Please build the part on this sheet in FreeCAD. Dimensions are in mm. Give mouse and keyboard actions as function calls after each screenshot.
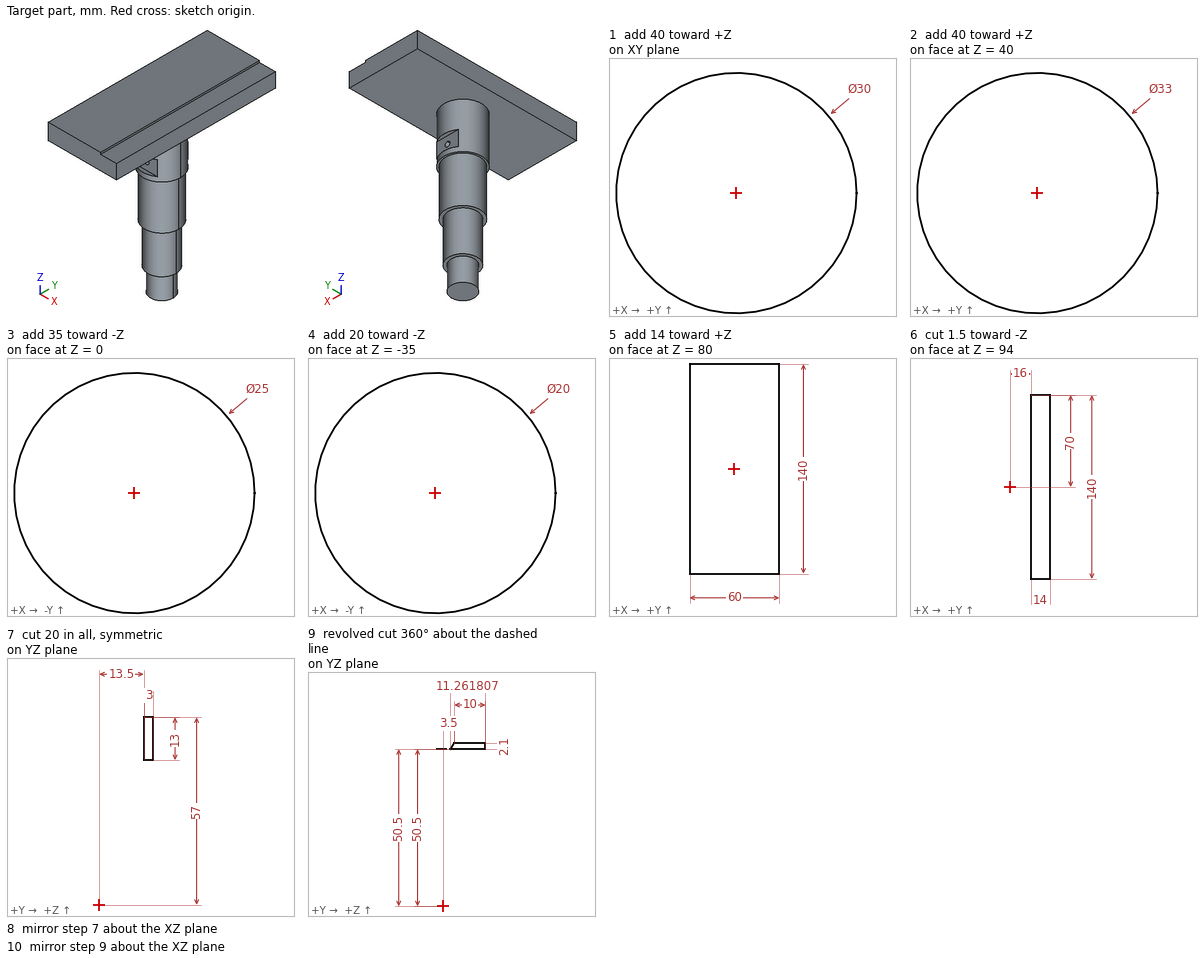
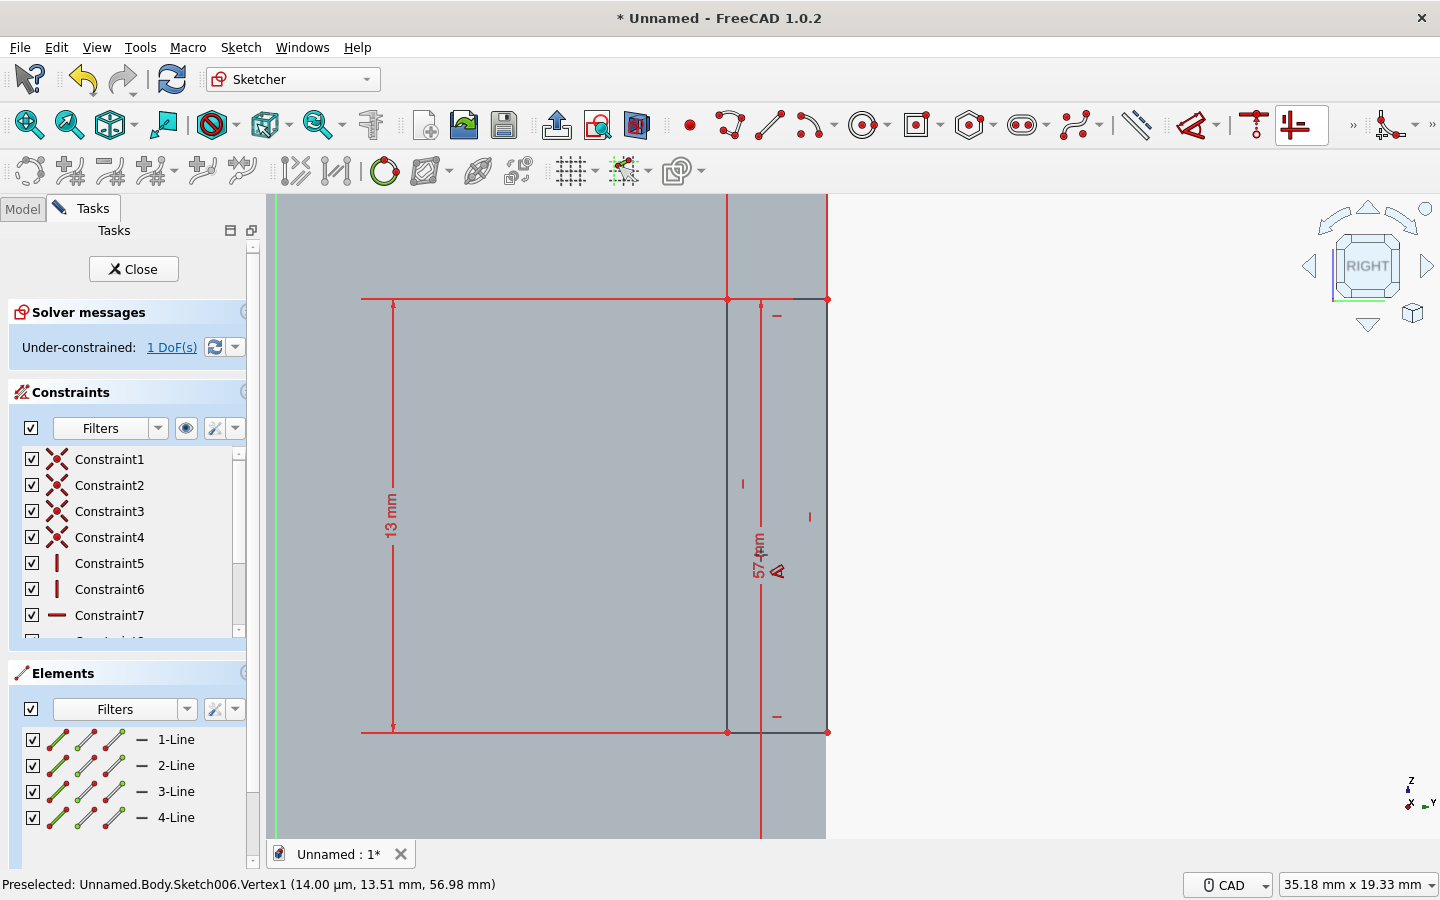
click(727, 299)
click(511, 265)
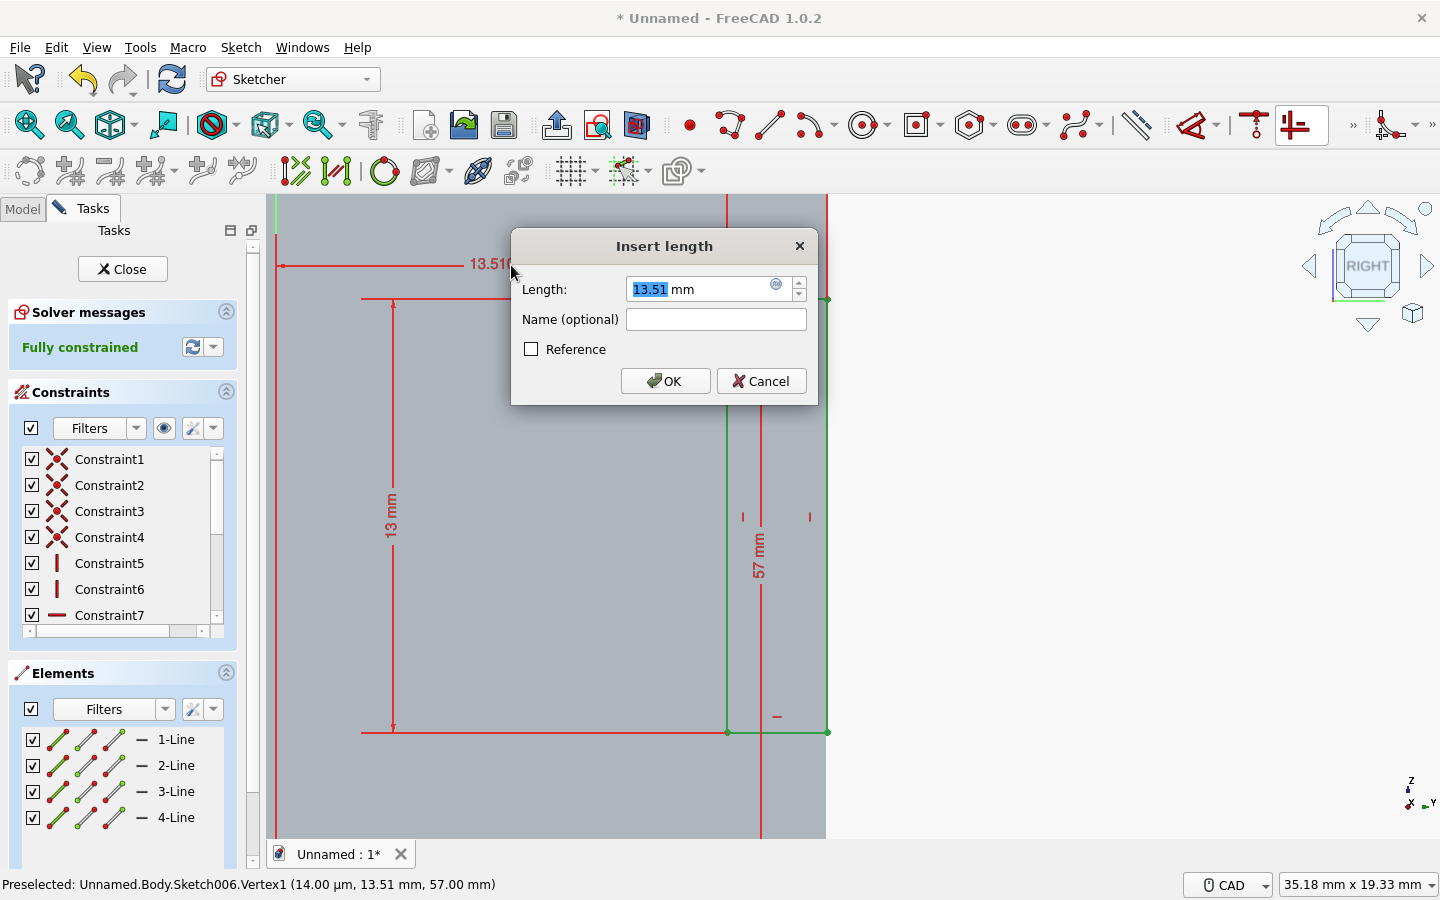
text(13.5)
key(Return)
key(Escape)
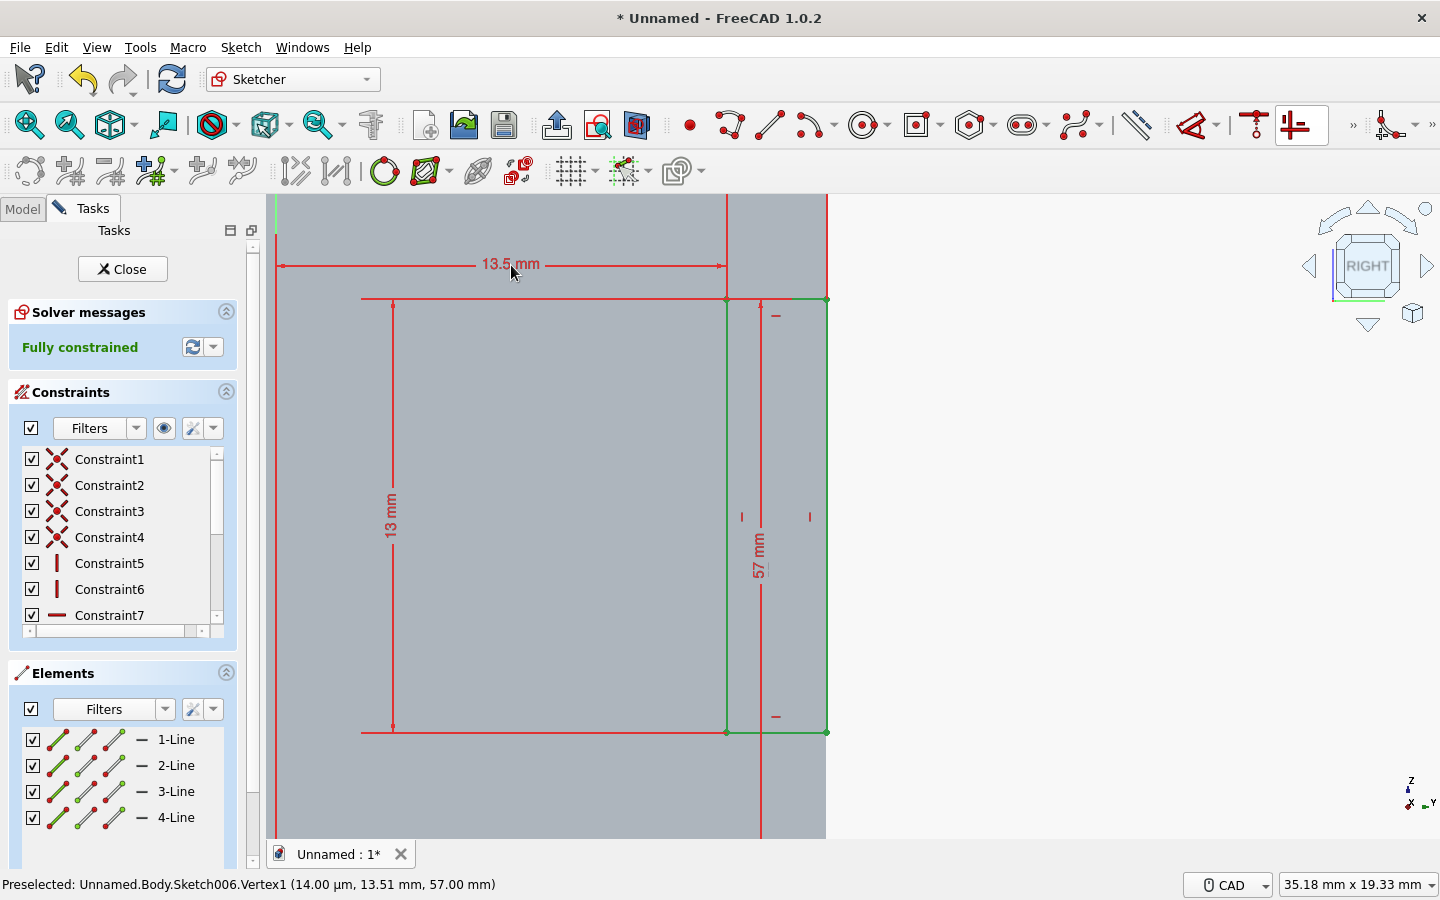
click(123, 269)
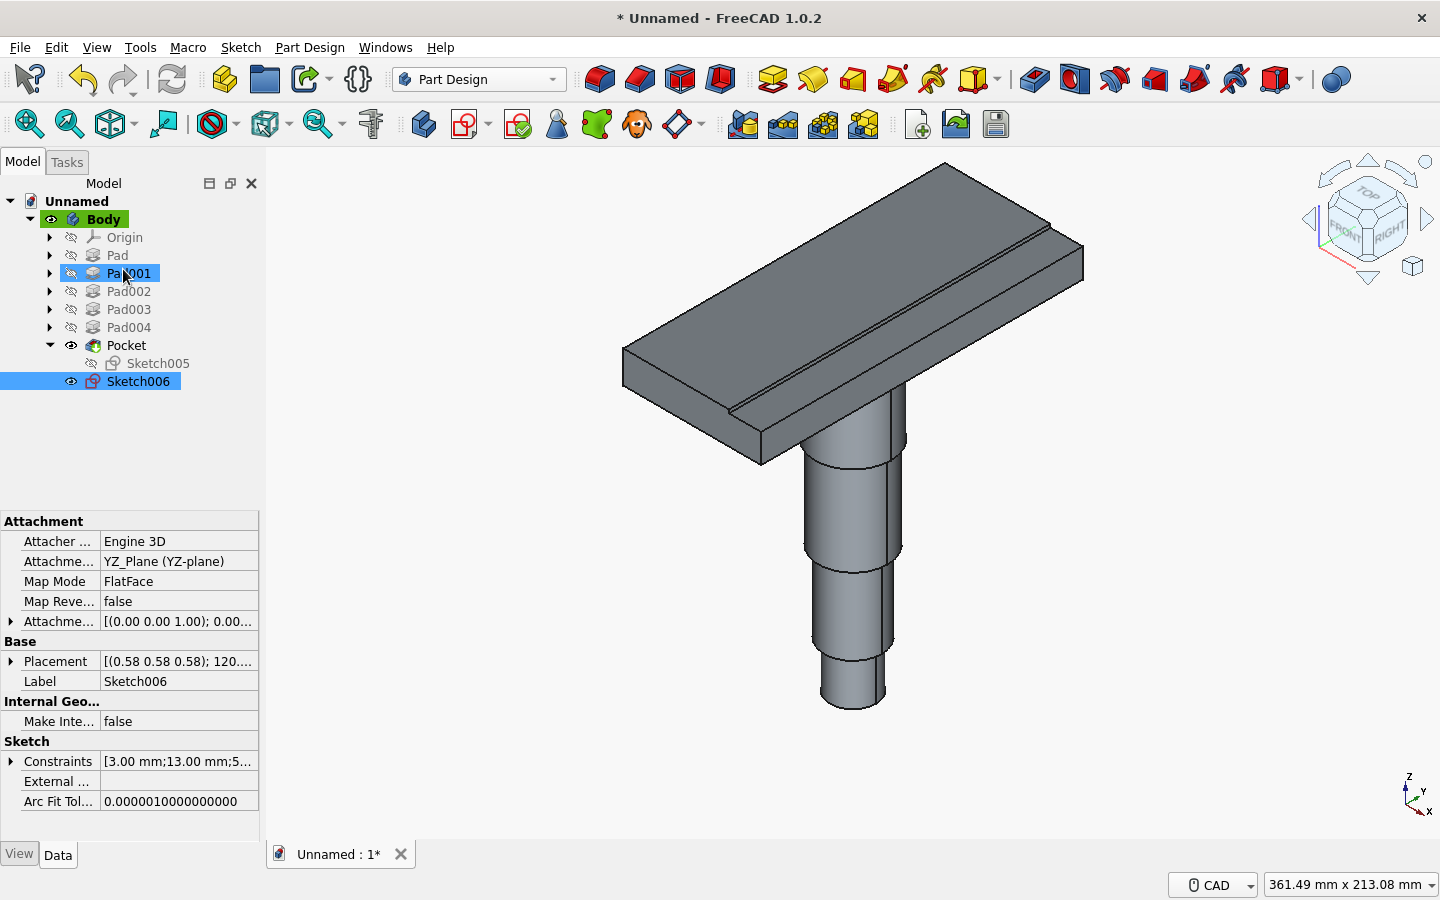
click(1036, 80)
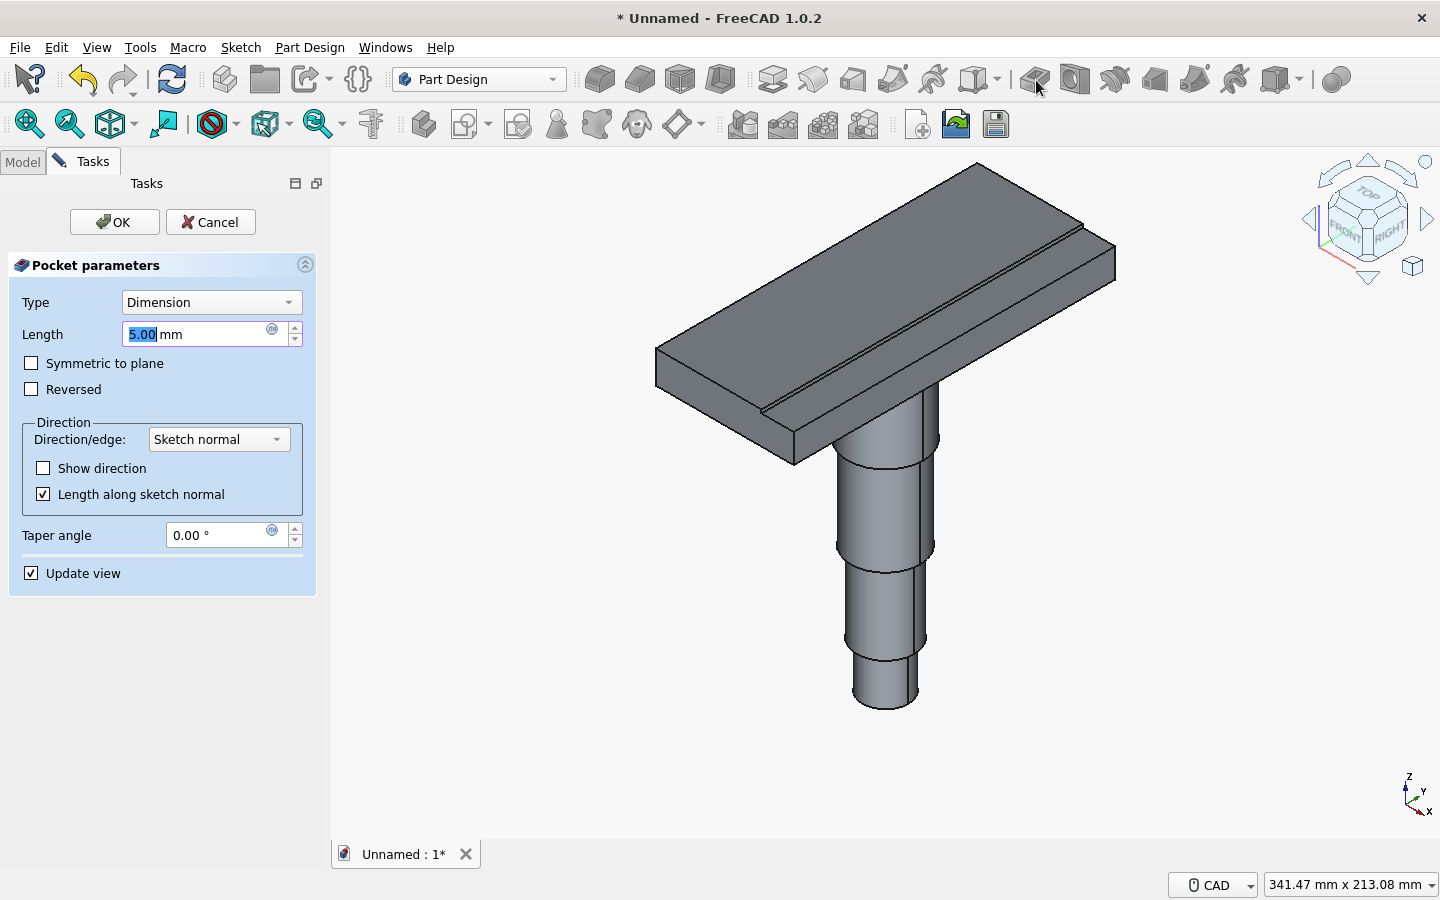
text(20)
key(Tab)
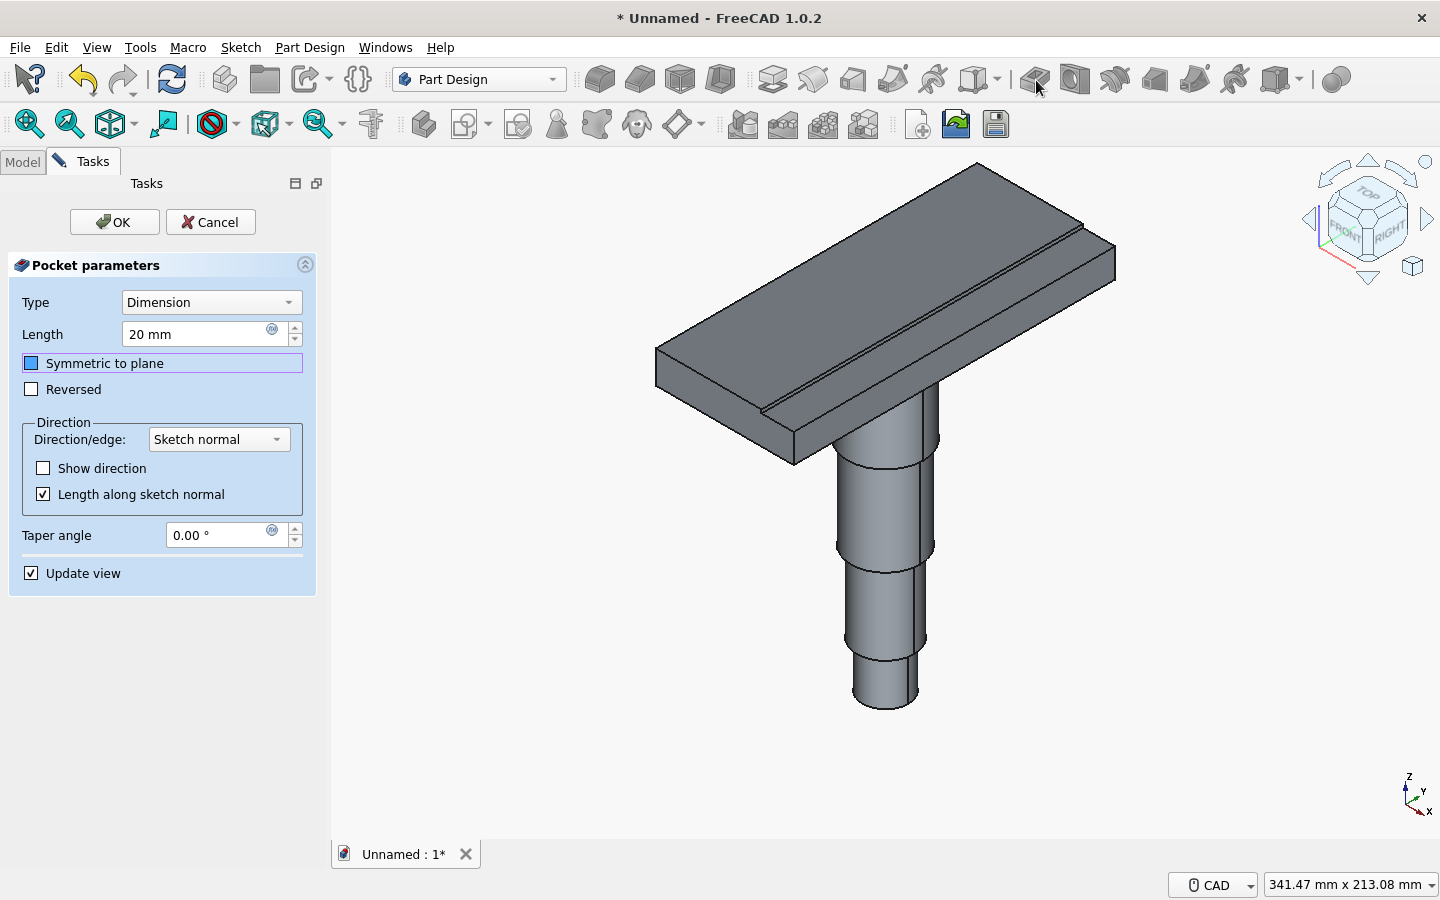
click(30, 363)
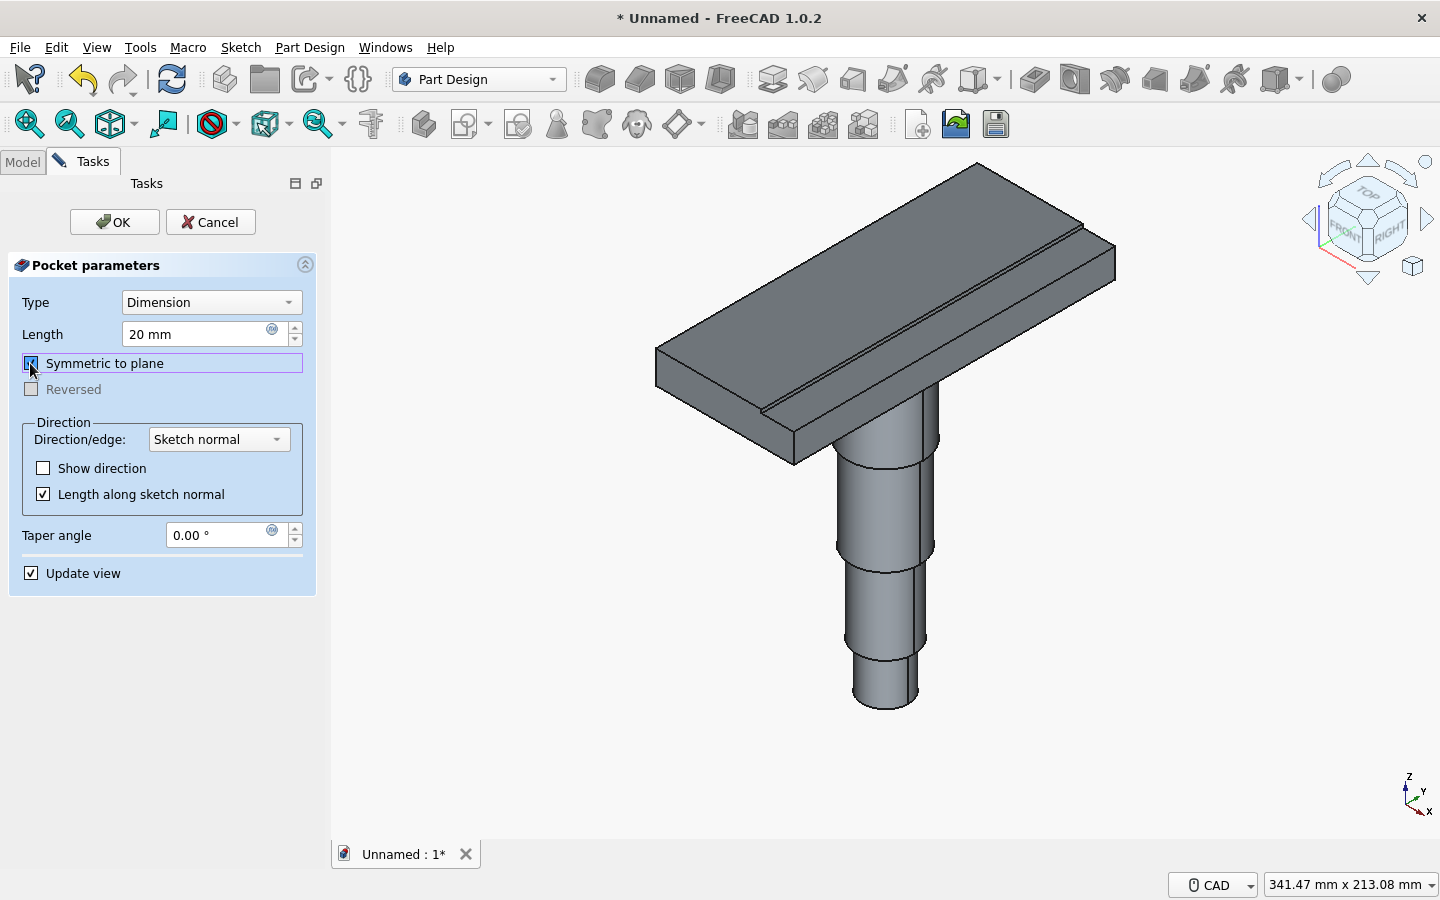
click(115, 222)